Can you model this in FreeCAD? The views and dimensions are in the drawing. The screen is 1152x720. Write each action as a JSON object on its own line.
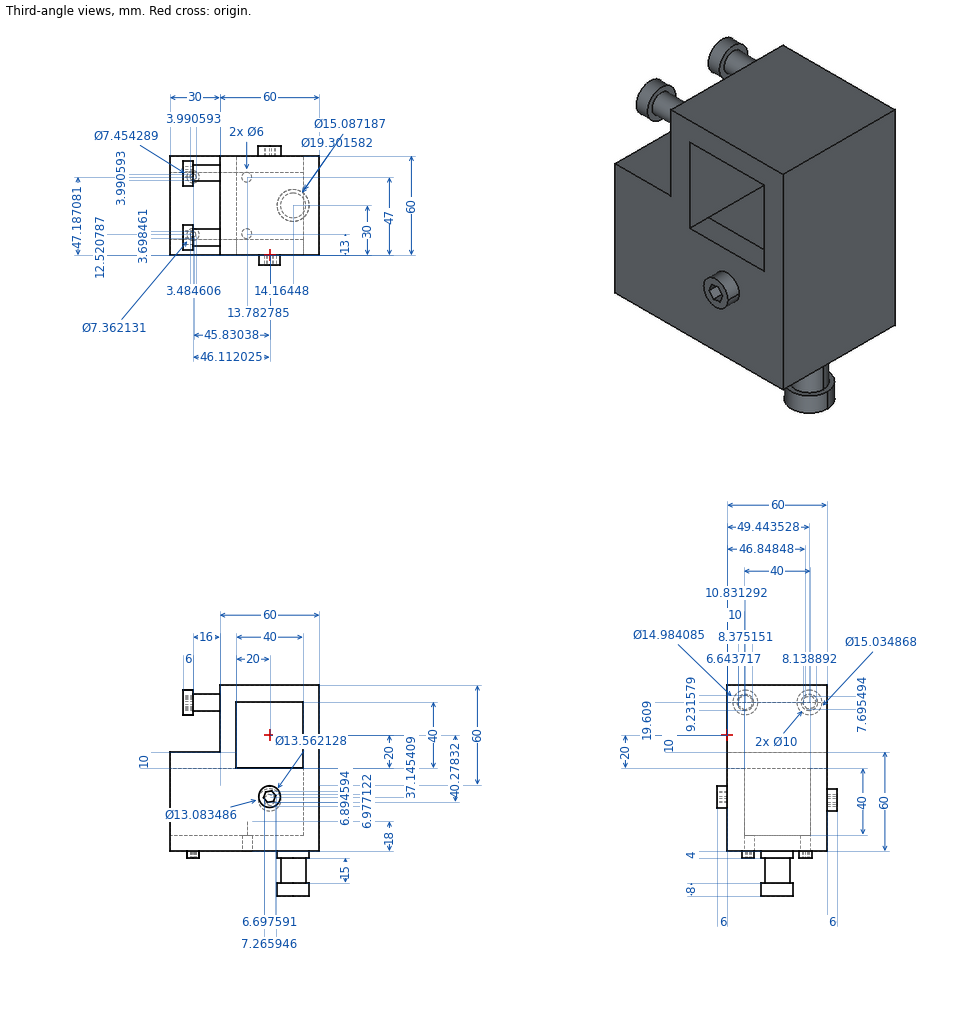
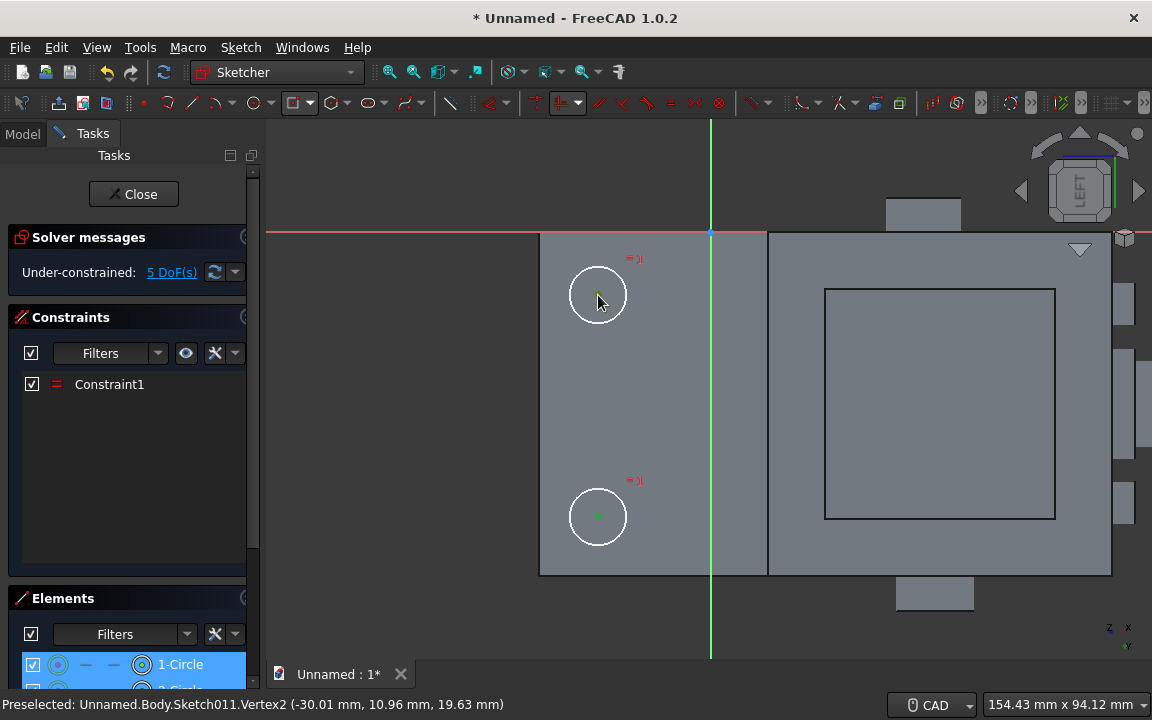
{"action": "left_click", "coordinate": [580, 104]}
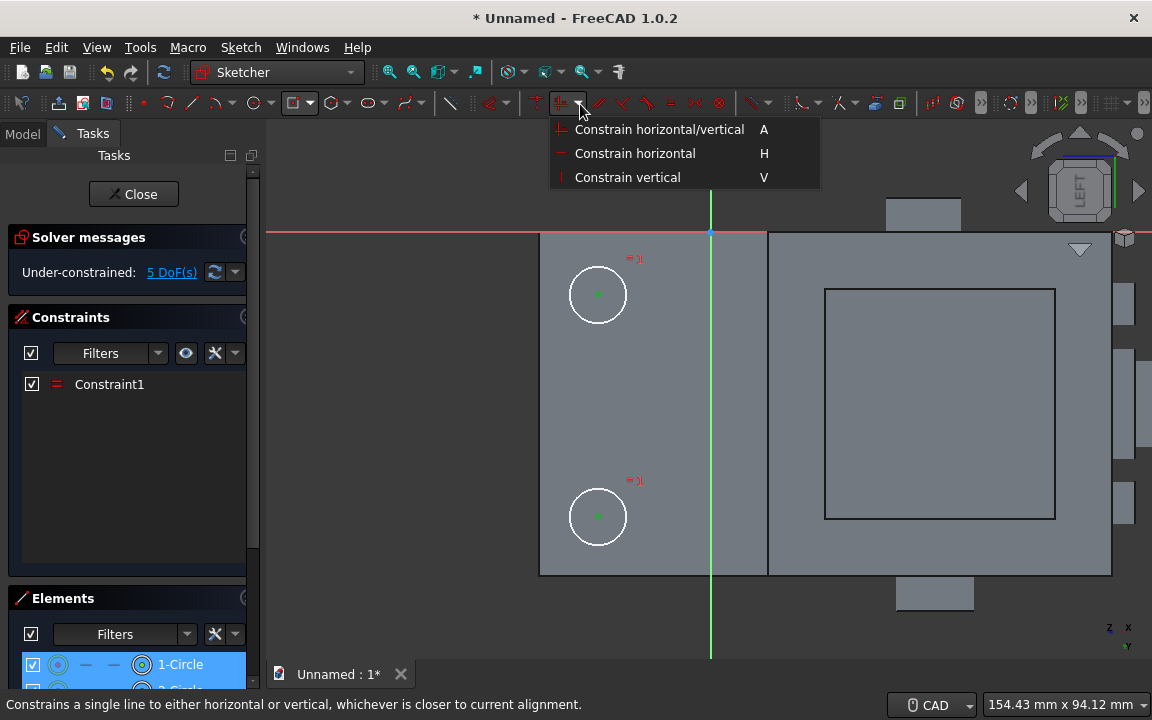
{"action": "left_click", "coordinate": [685, 177]}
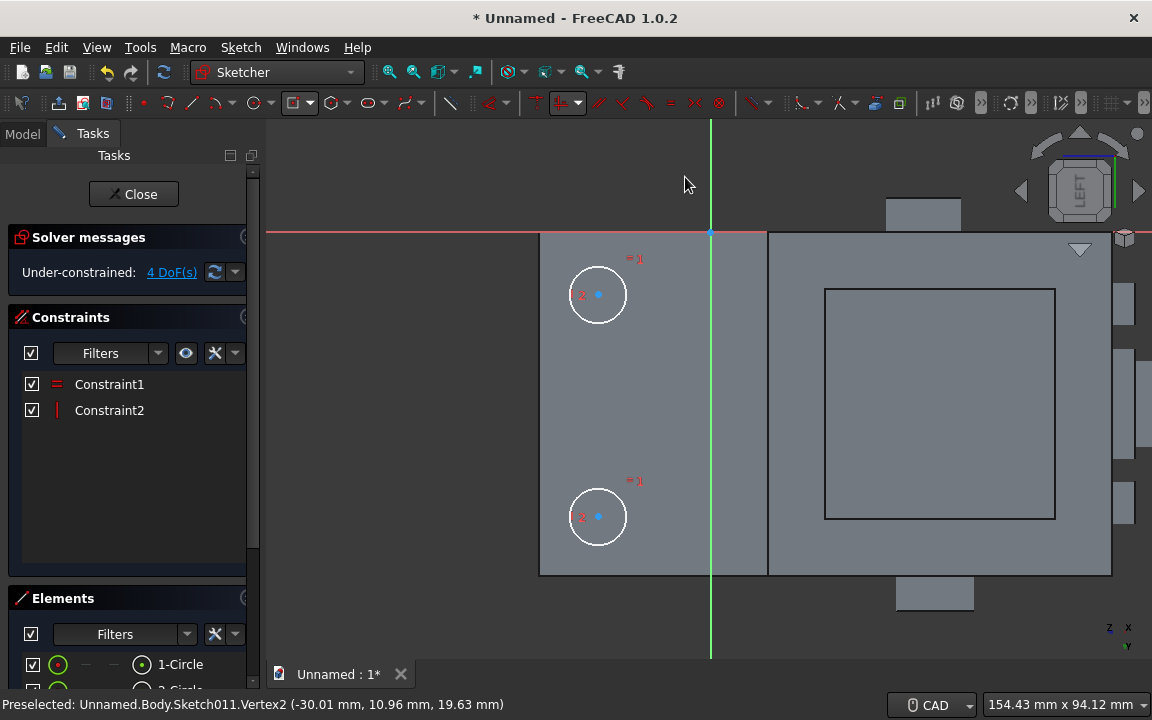
{"action": "left_click", "coordinate": [490, 104]}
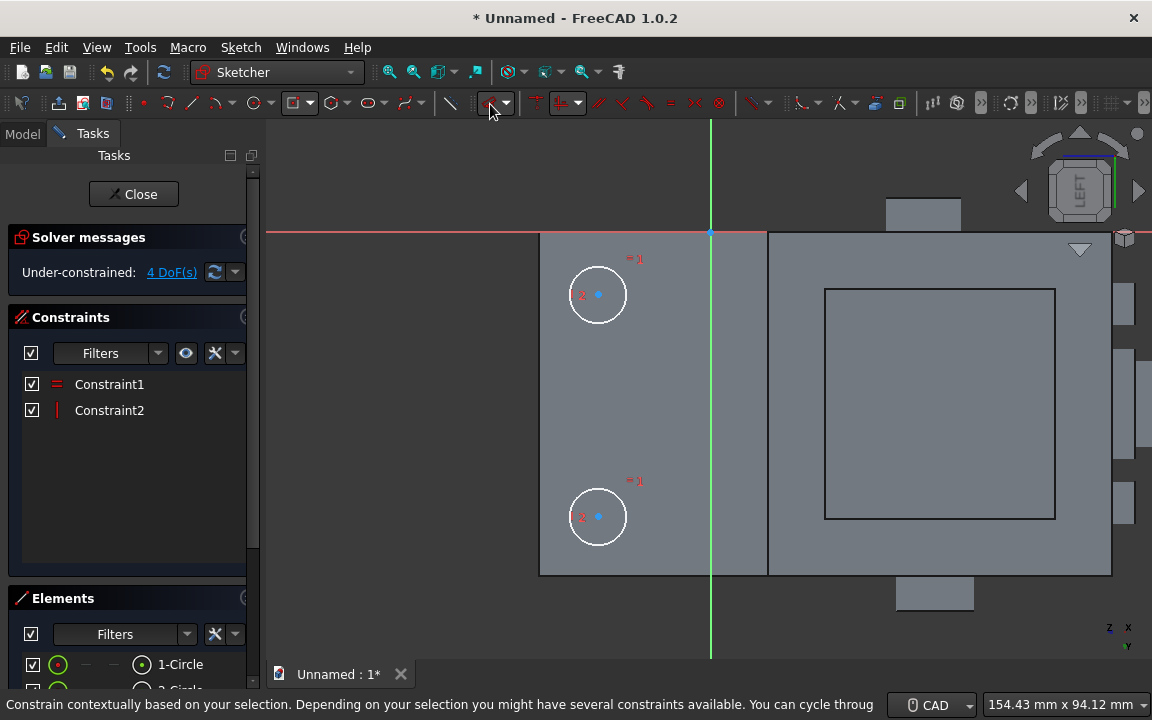
{"action": "left_click", "coordinate": [618, 497]}
{"action": "left_click", "coordinate": [641, 474]}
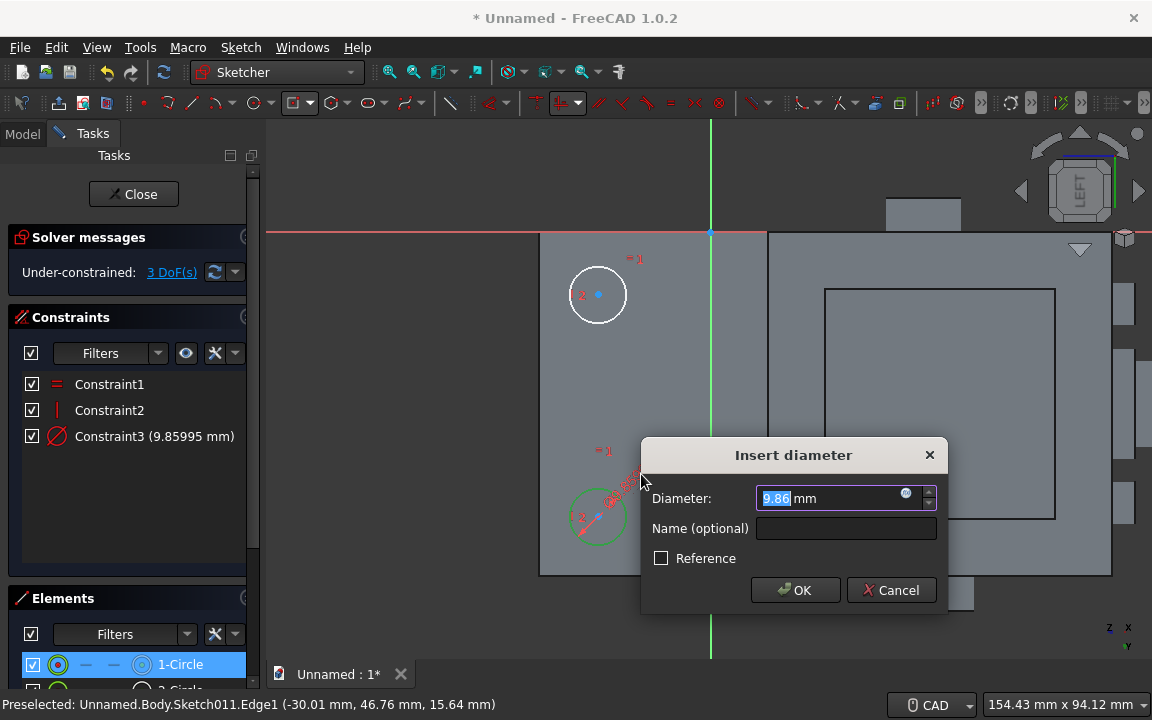
{"action": "type", "text": "10"}
{"action": "key", "text": "Return"}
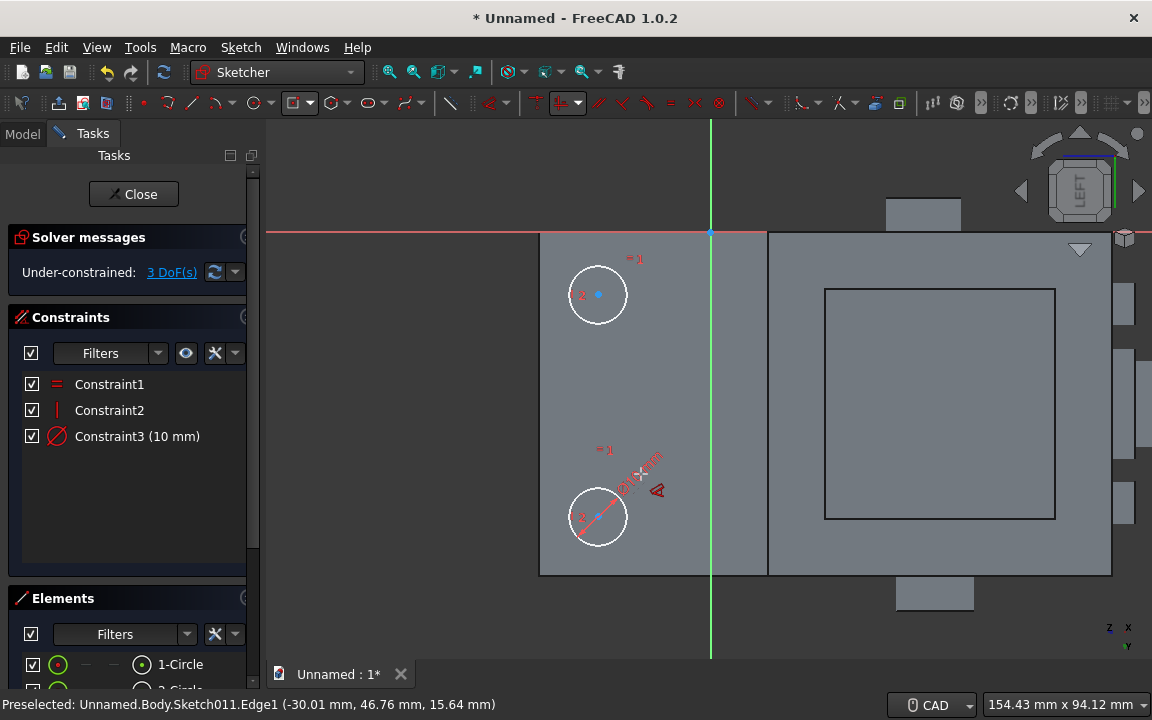
{"action": "left_click", "coordinate": [598, 517]}
{"action": "left_click", "coordinate": [654, 198]}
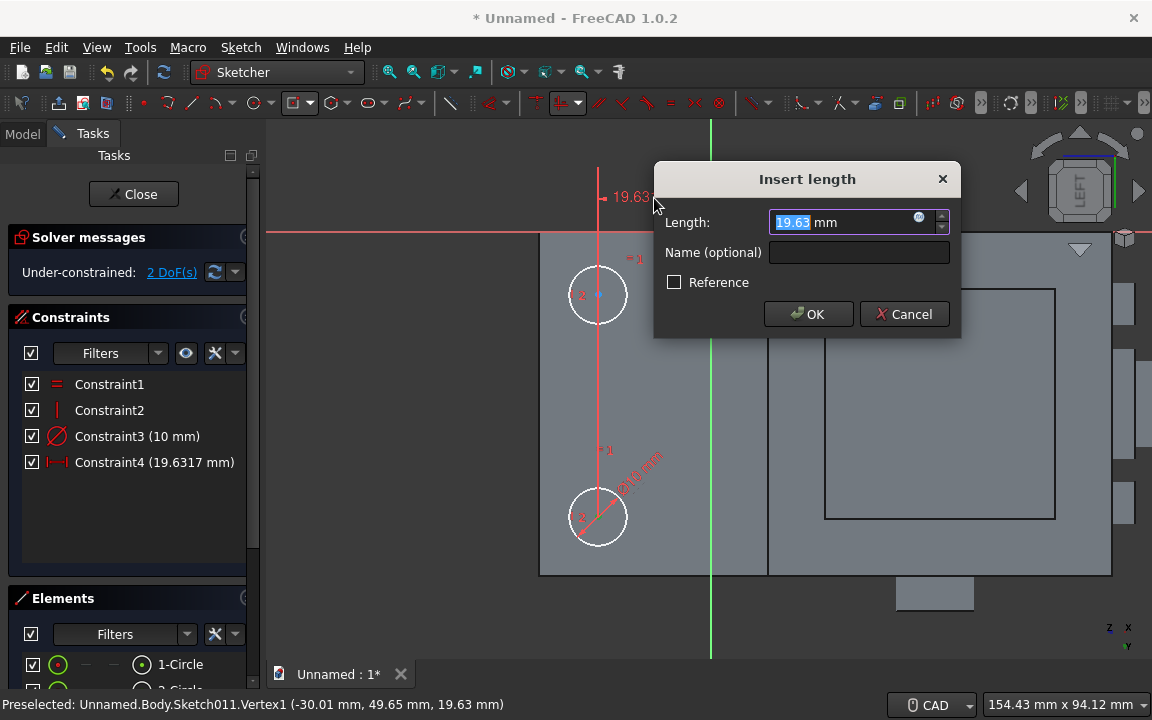
{"action": "type", "text": "19.609"}
{"action": "key", "text": "Return"}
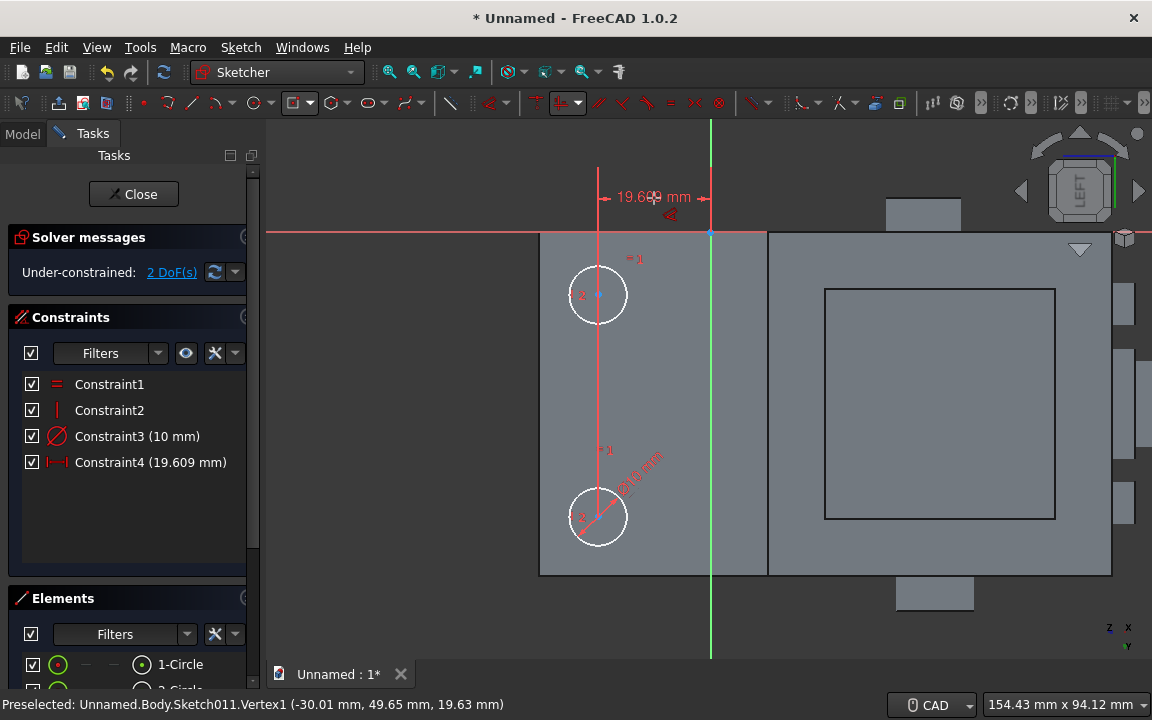
{"action": "left_click", "coordinate": [598, 517]}
{"action": "left_click", "coordinate": [745, 375]}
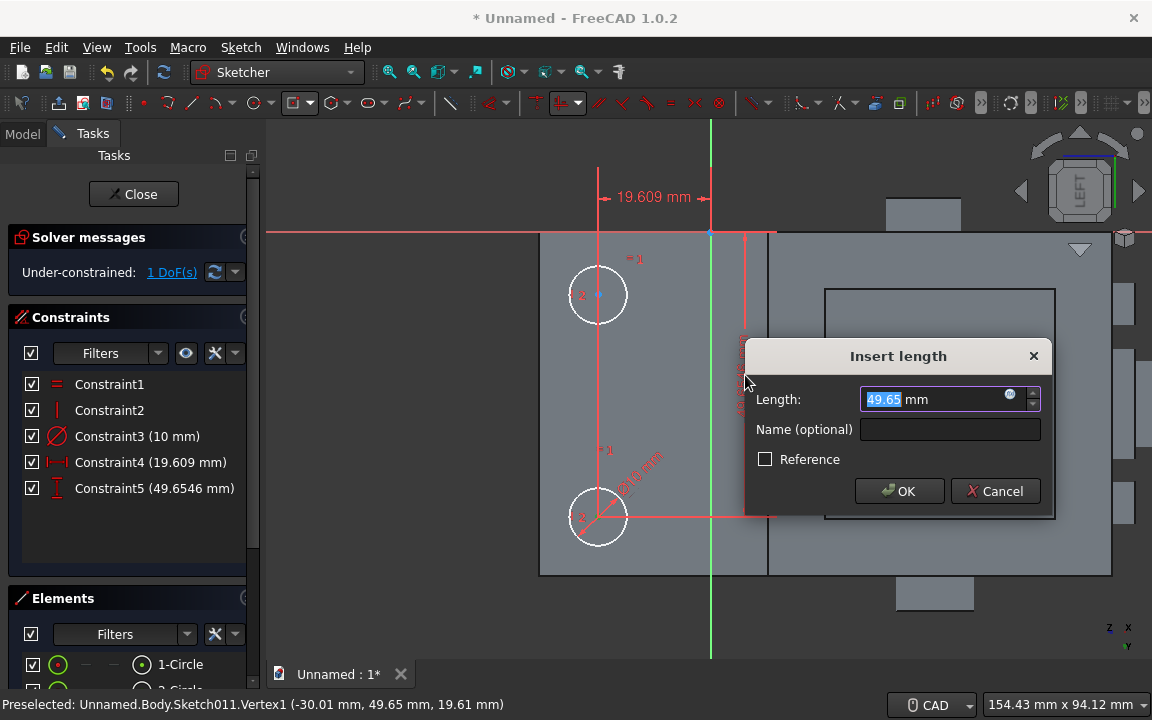
{"action": "type", "text": "49.443528"}
{"action": "key", "text": "Return"}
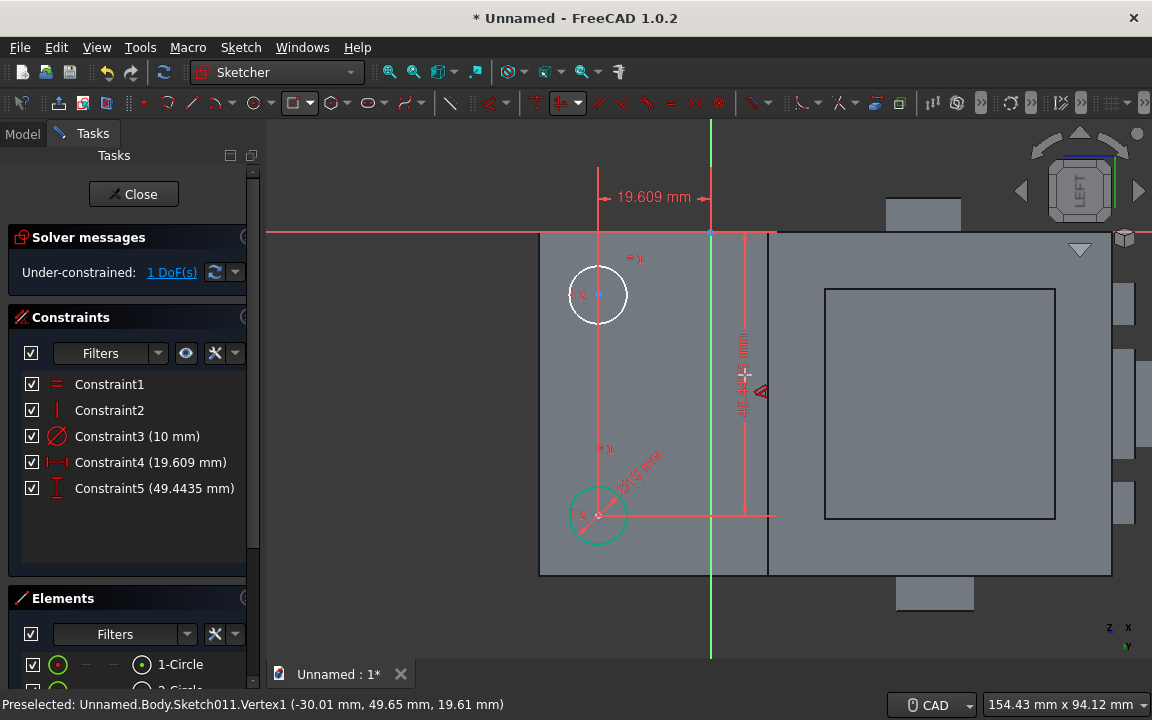
{"action": "left_click", "coordinate": [598, 295]}
{"action": "left_click", "coordinate": [745, 264]}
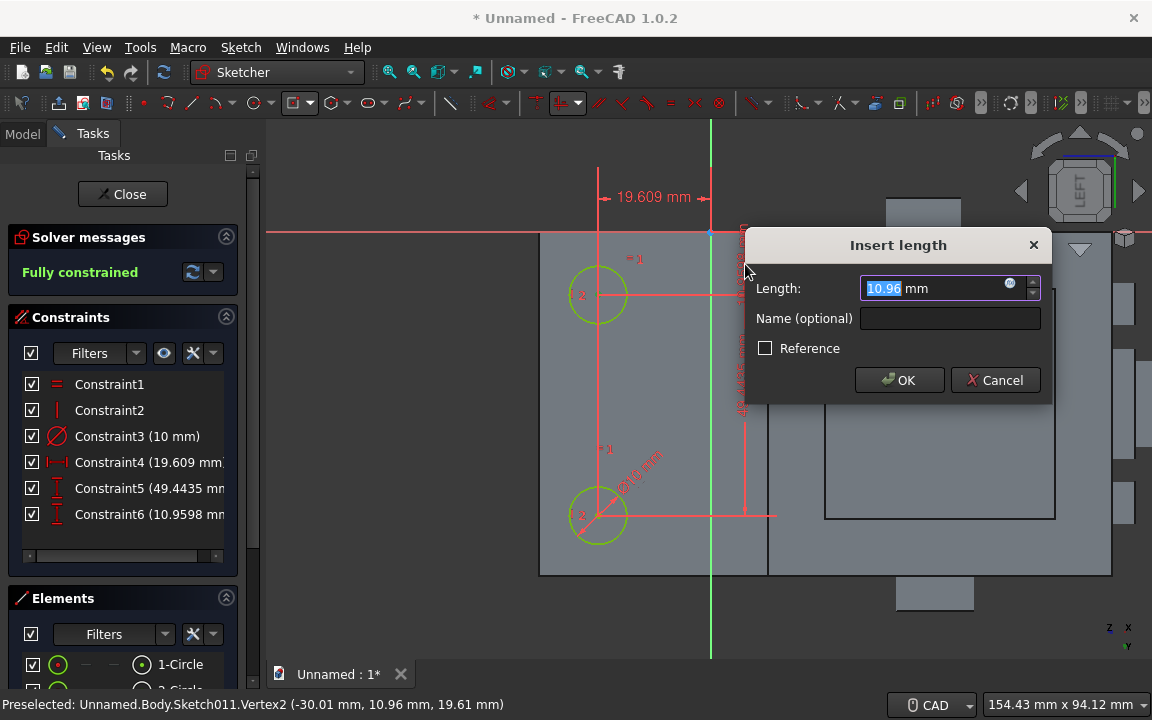
{"action": "type", "text": "10.831292"}
{"action": "key", "text": "Return"}
{"action": "key", "text": "Escape"}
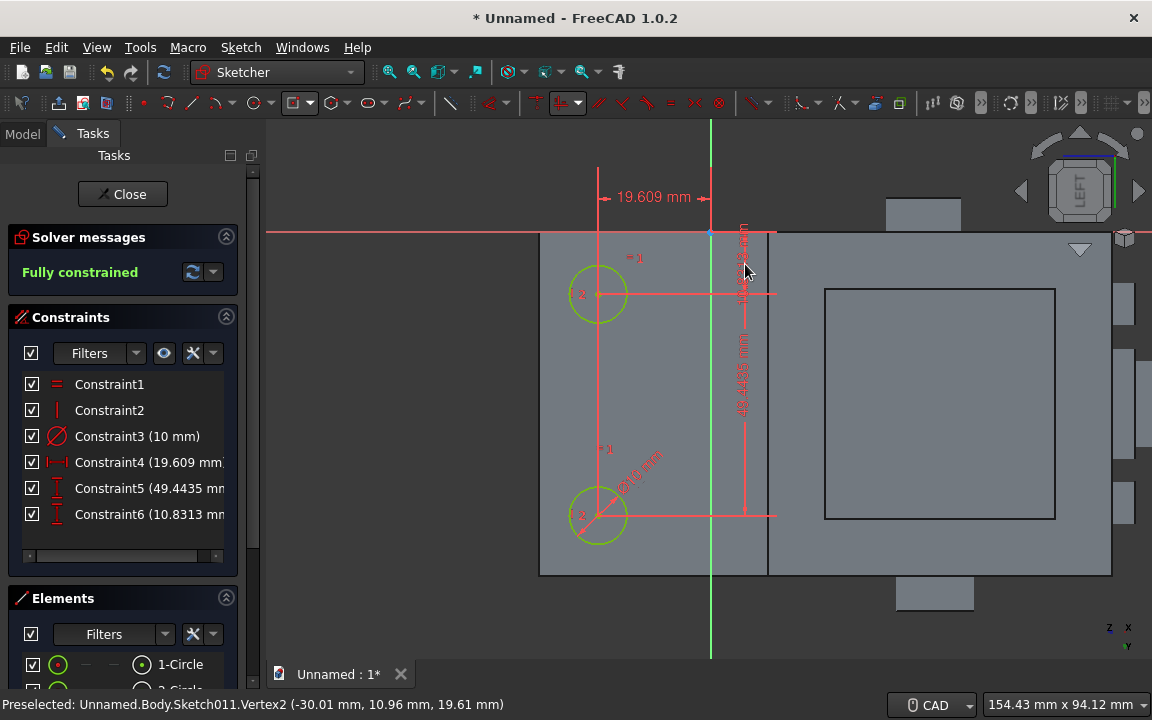
{"action": "left_click", "coordinate": [123, 194]}